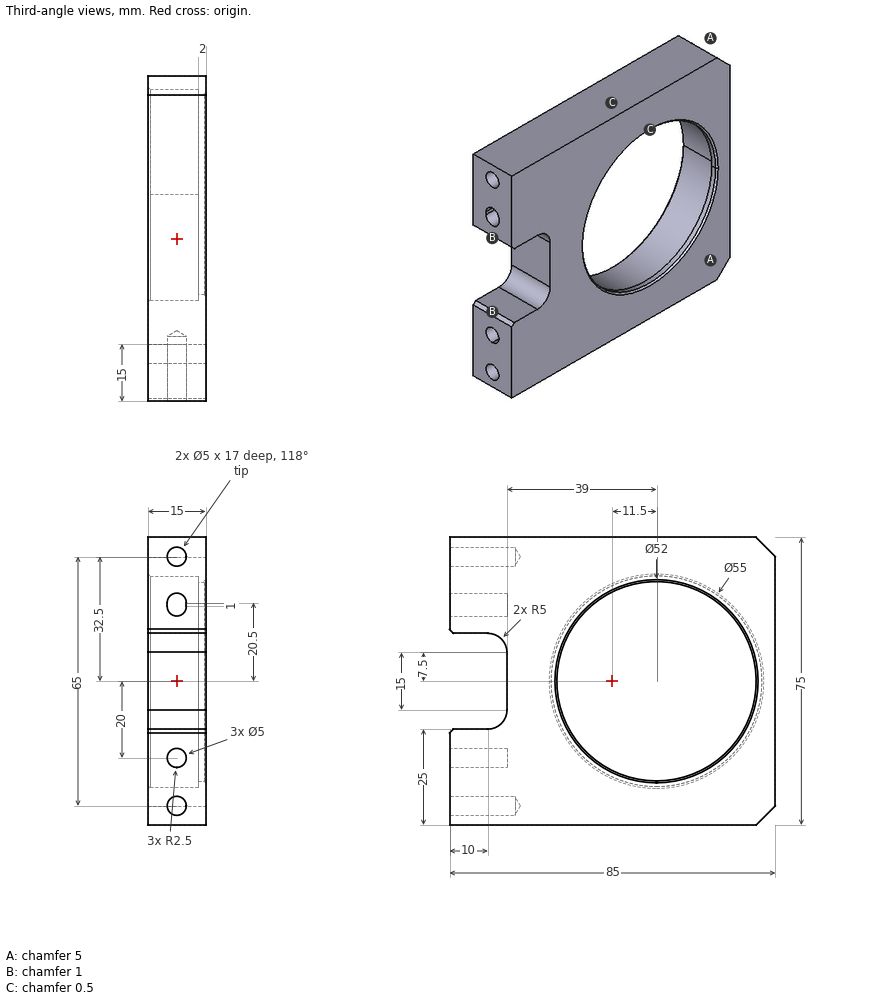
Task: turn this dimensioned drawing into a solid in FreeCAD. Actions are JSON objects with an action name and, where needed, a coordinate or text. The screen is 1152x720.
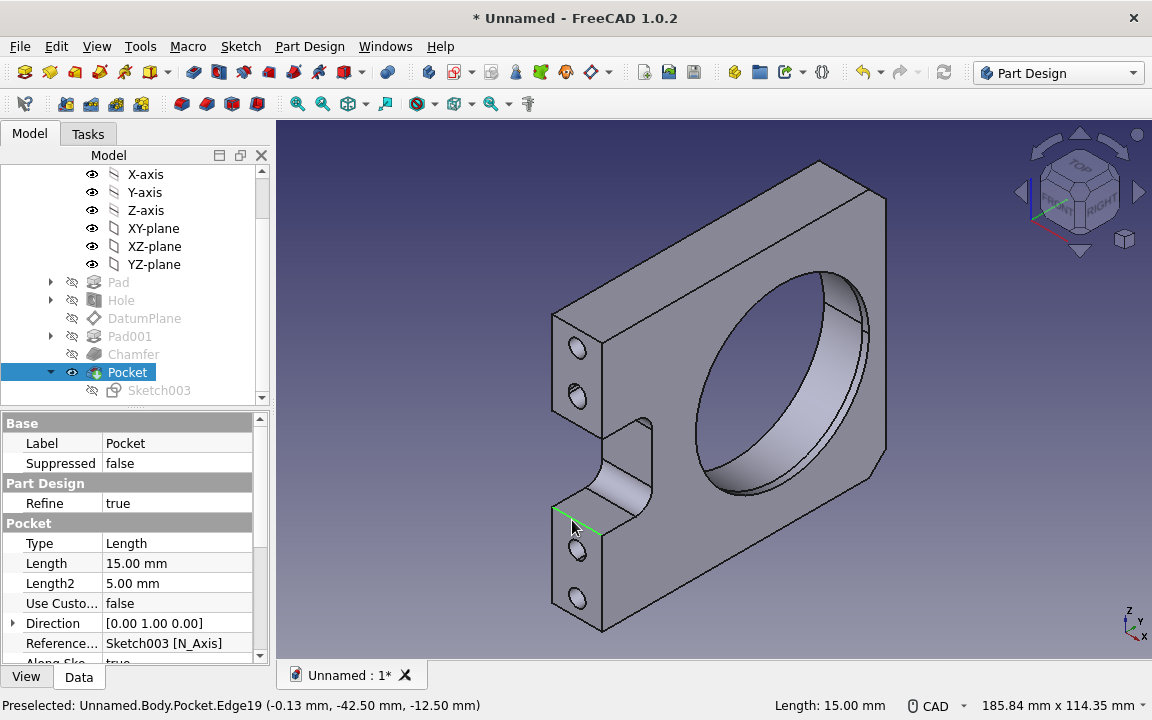
{"action": "key", "text": "2"}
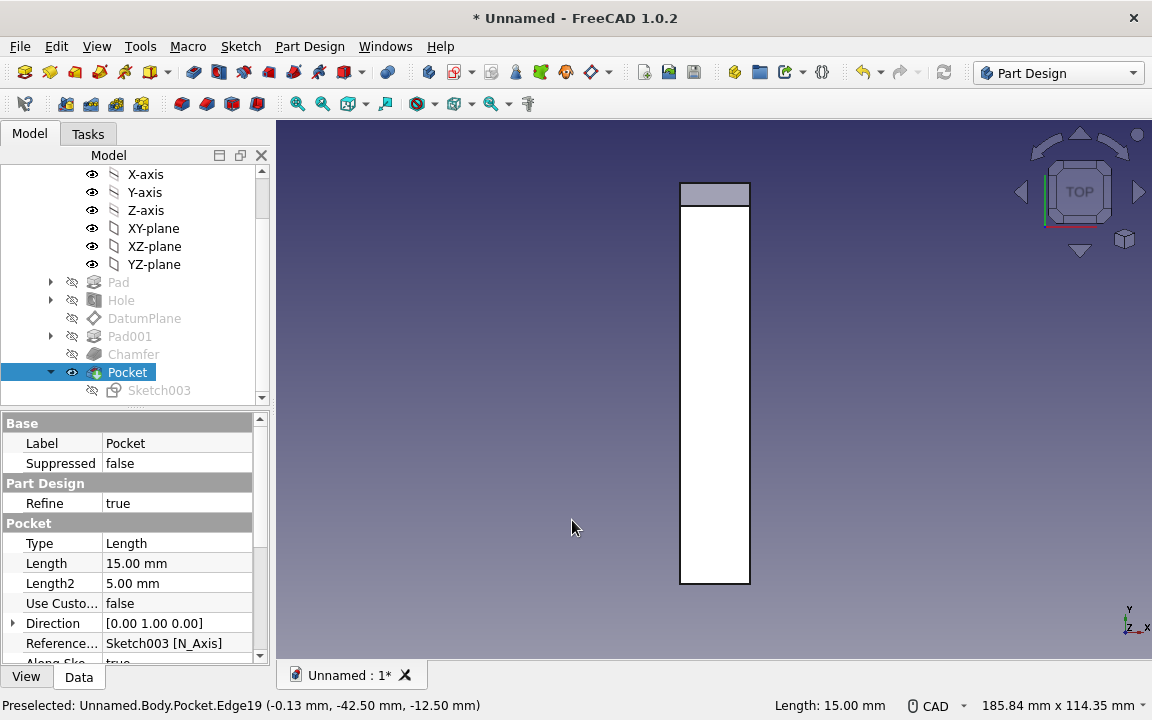
{"action": "key", "text": "0"}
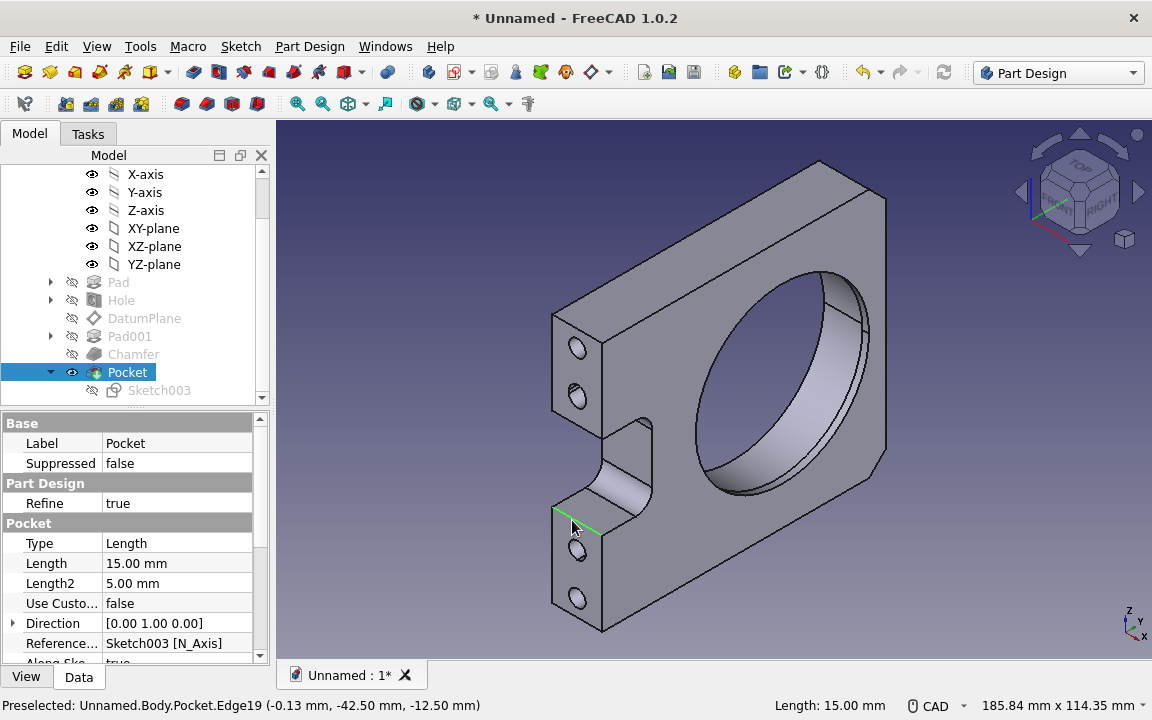
{"action": "key", "text": "1"}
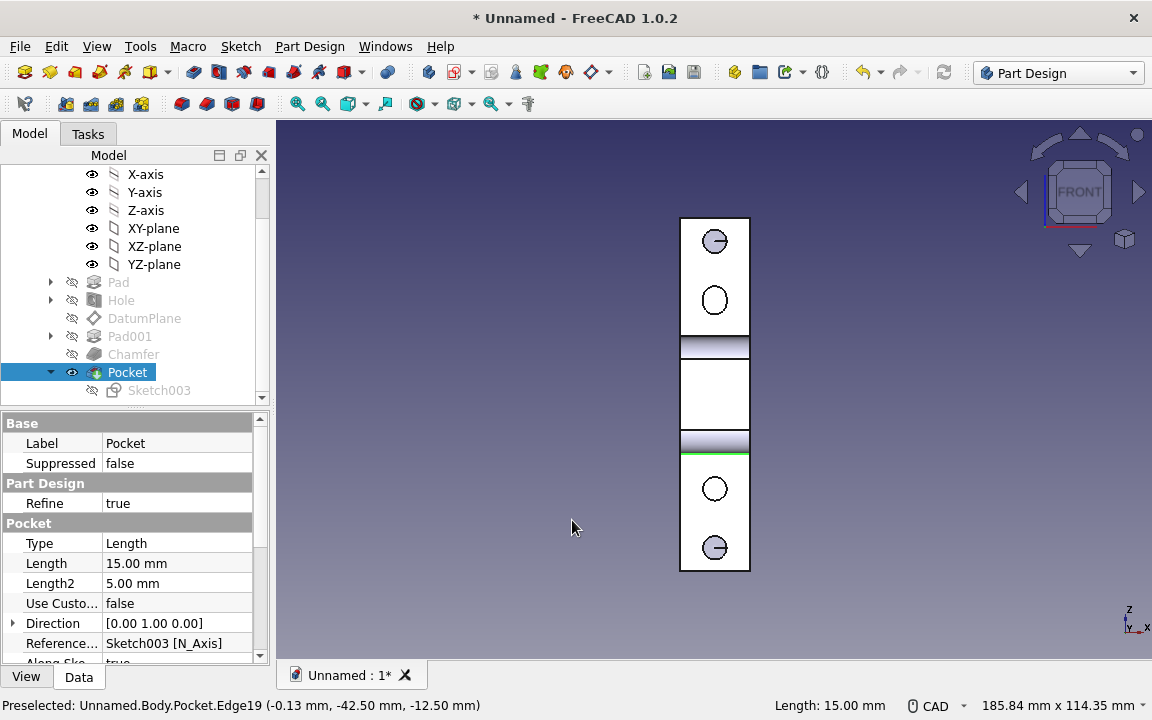
{"action": "left_click", "coordinate": [715, 335], "text": "ctrl"}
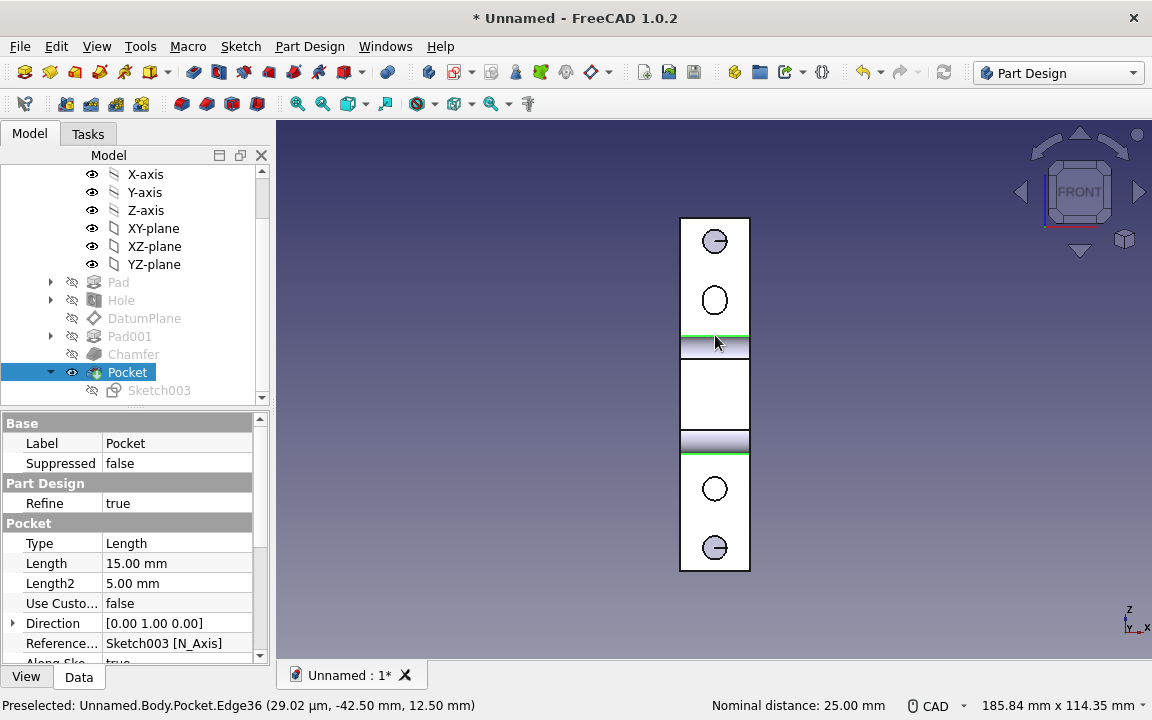
{"action": "left_click", "coordinate": [207, 104]}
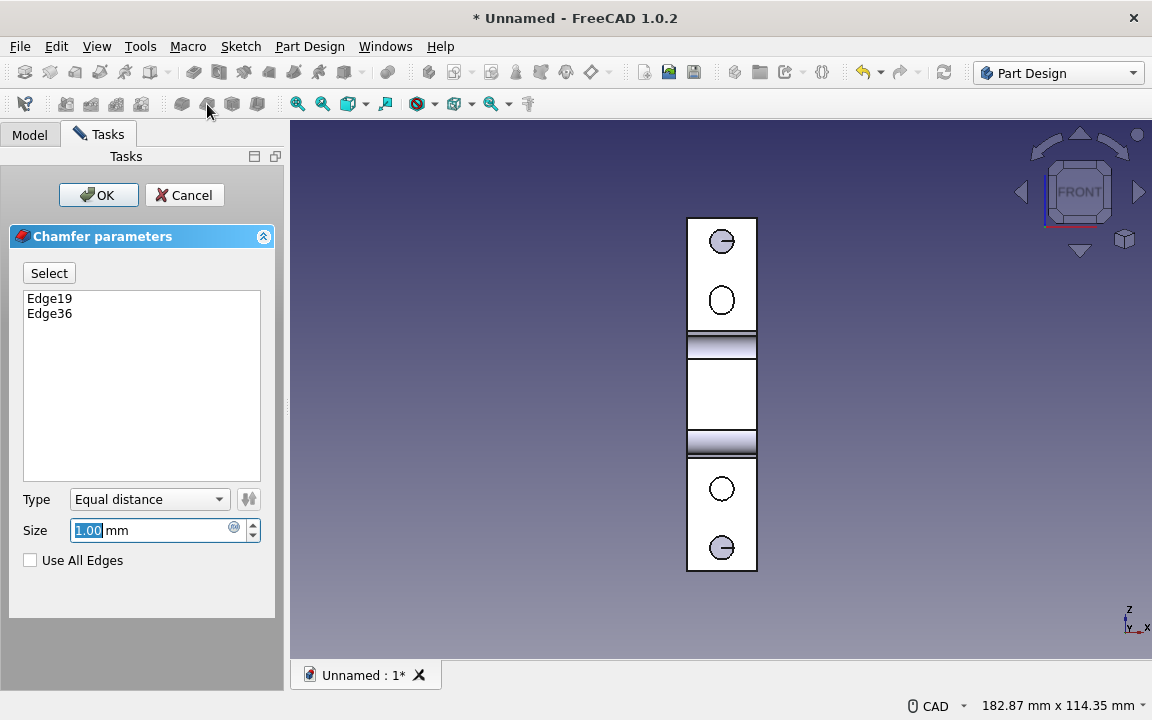
{"action": "type", "text": "1"}
{"action": "key", "text": "Tab"}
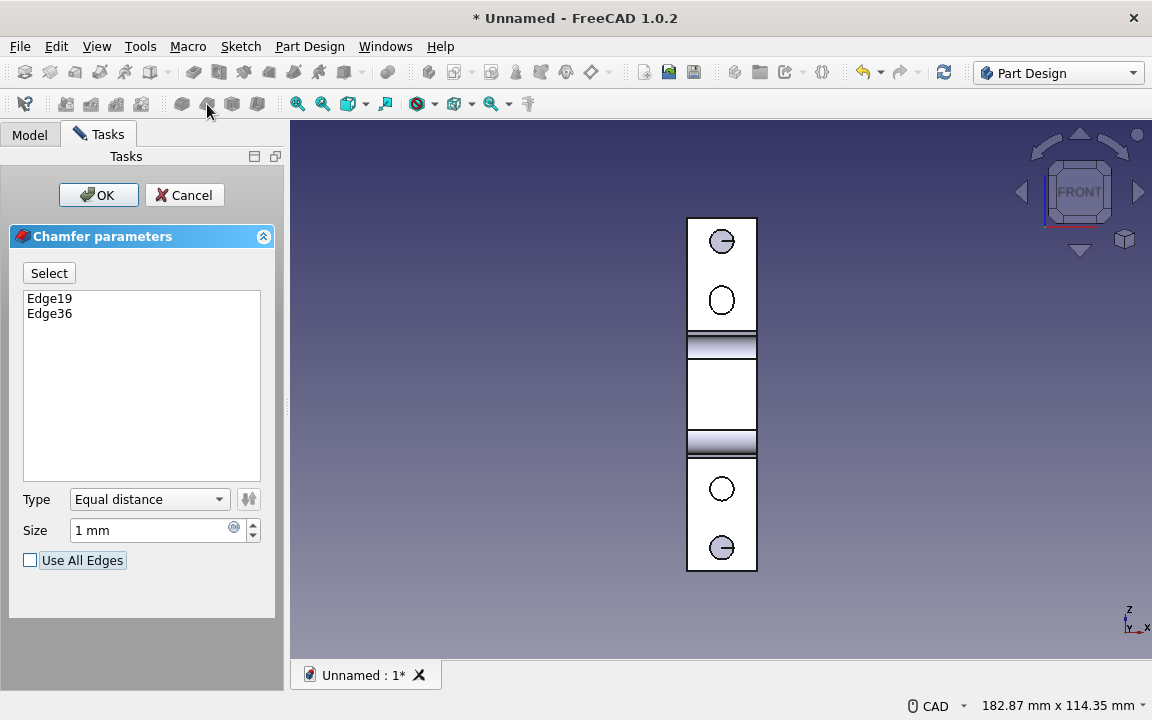
{"action": "left_click", "coordinate": [99, 195]}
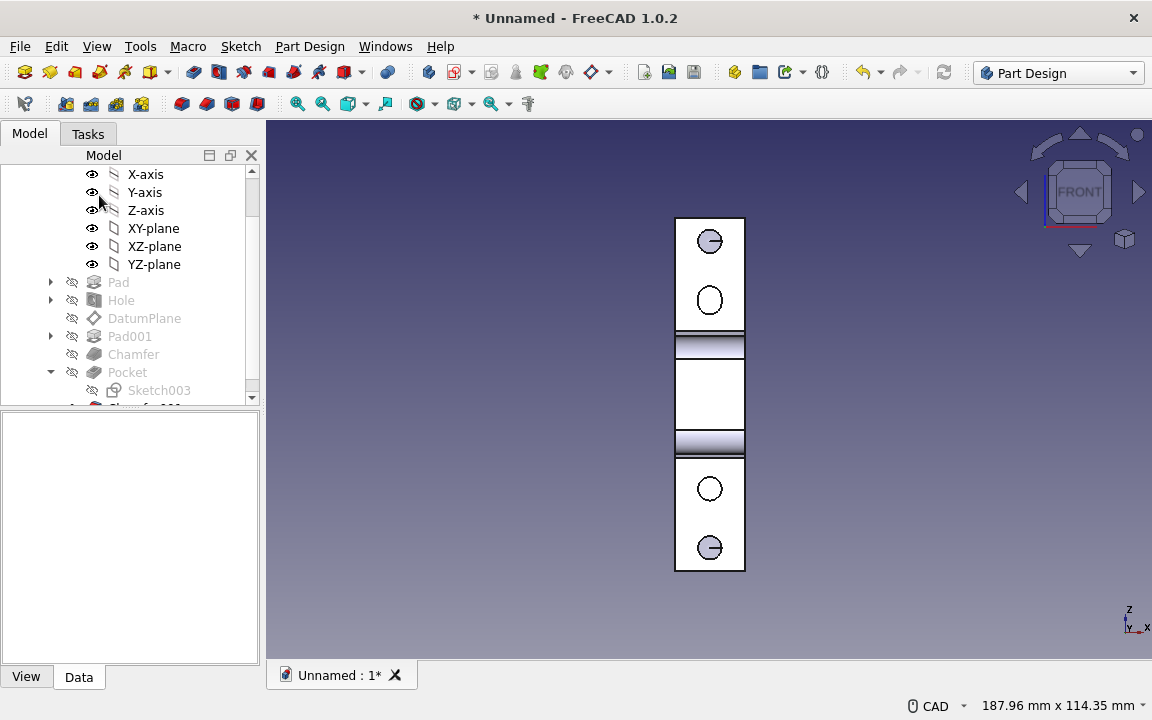
{"action": "key", "text": "0"}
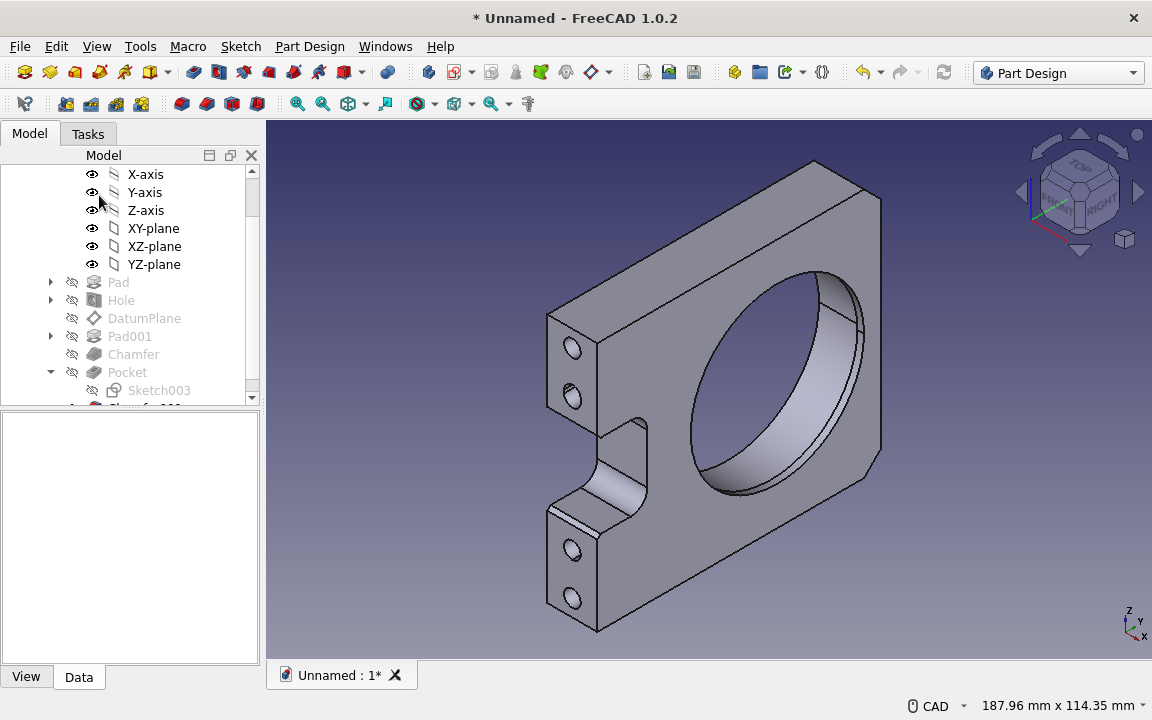
{"action": "left_click", "coordinate": [751, 493]}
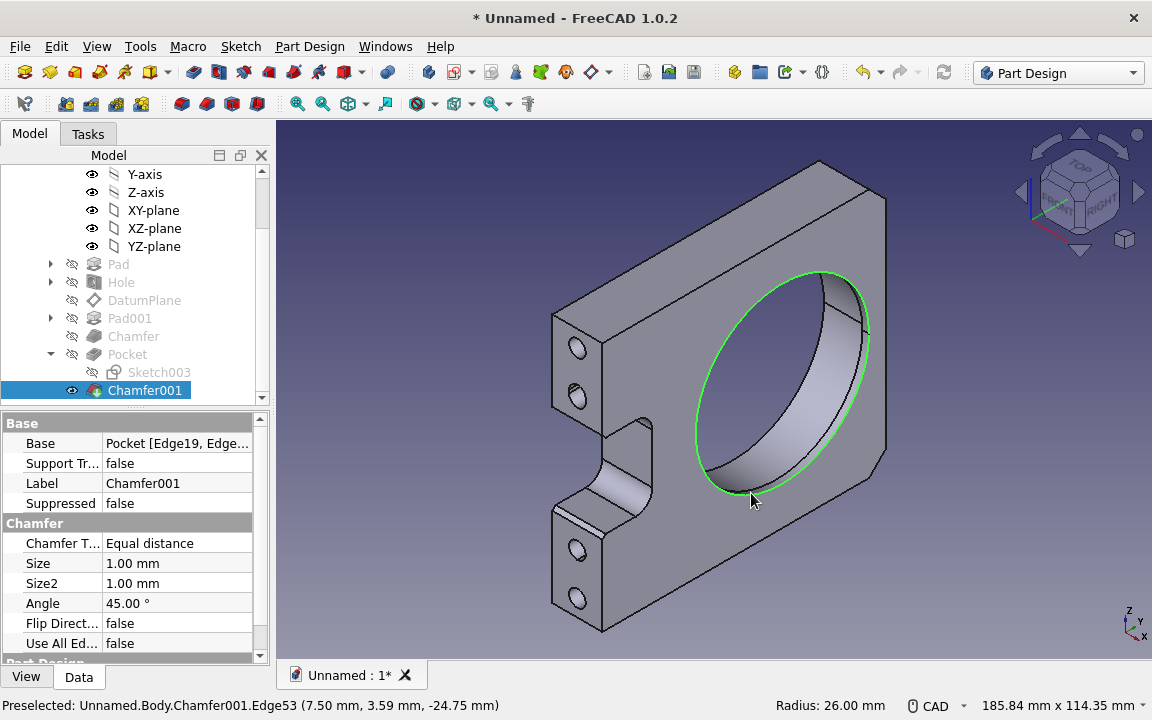
{"action": "key", "text": "2"}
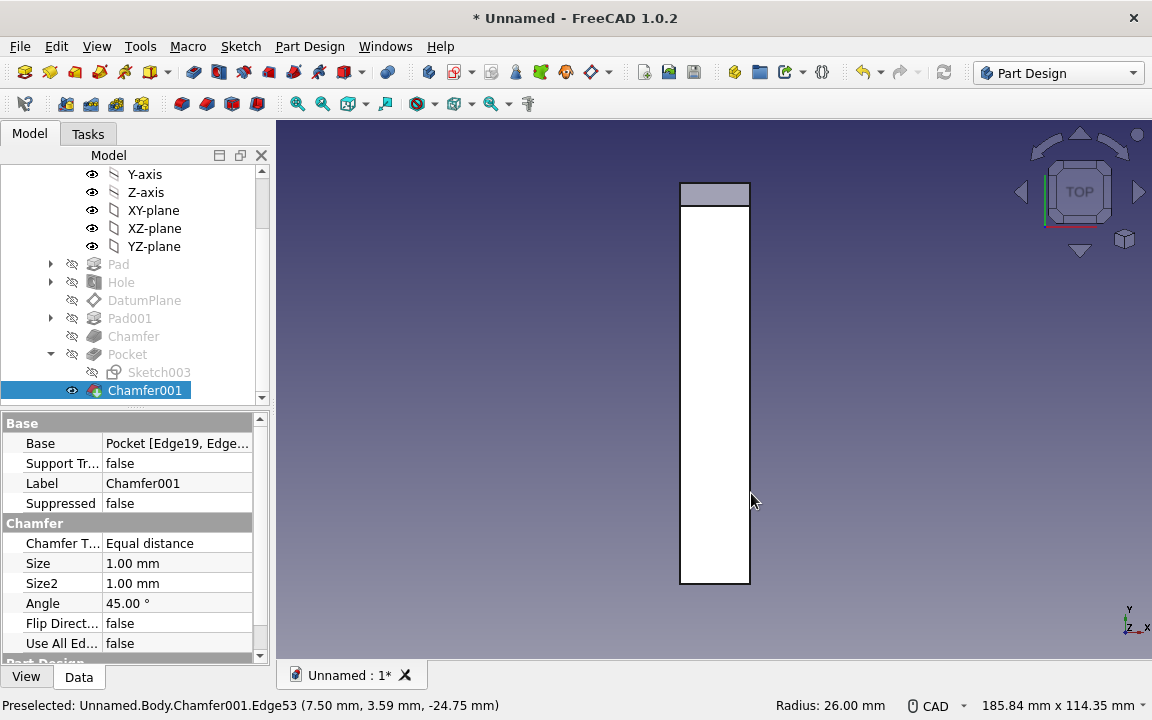
{"action": "key", "text": "1"}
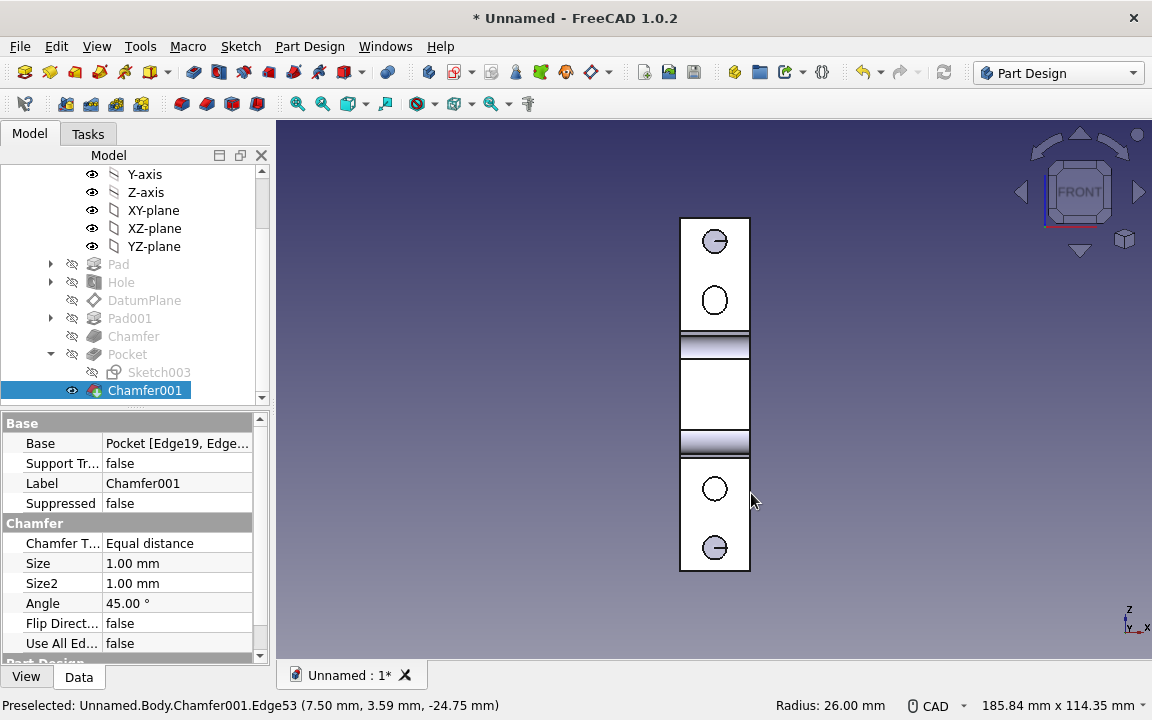
{"action": "key", "text": "3"}